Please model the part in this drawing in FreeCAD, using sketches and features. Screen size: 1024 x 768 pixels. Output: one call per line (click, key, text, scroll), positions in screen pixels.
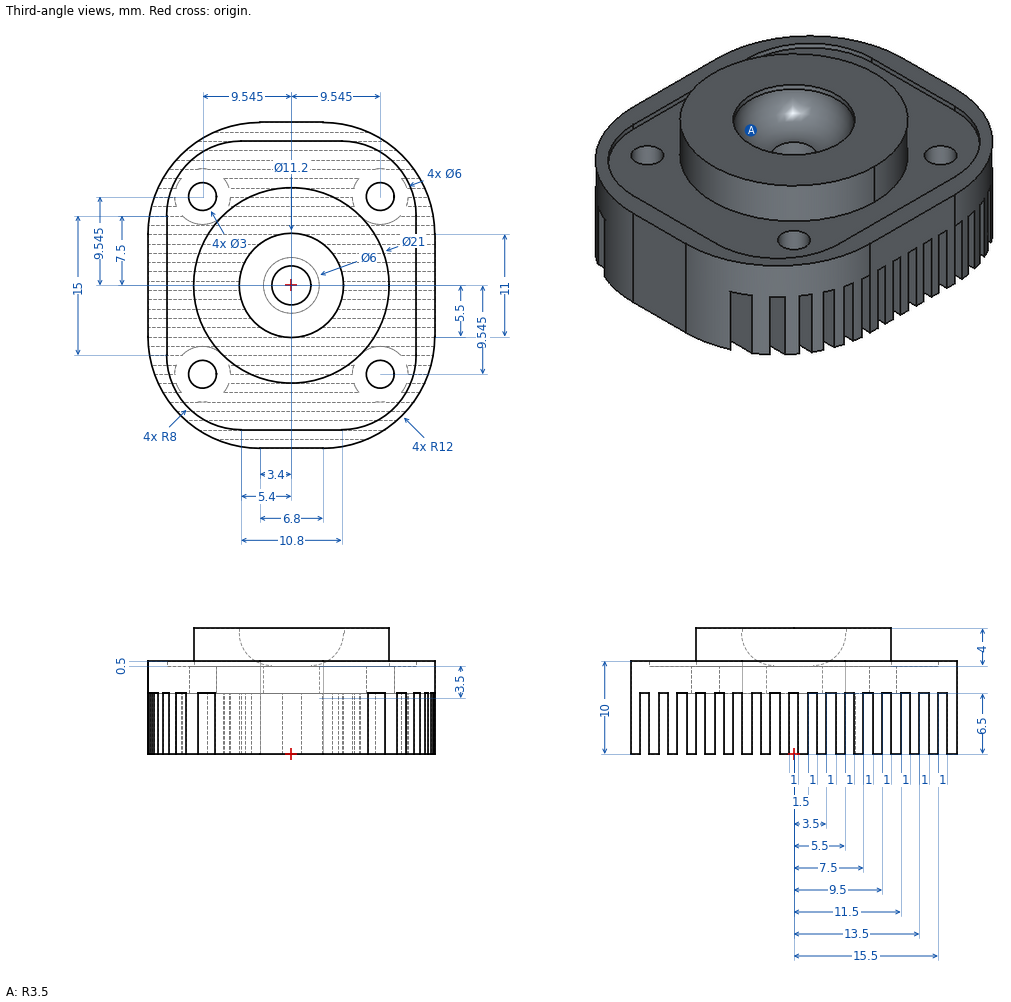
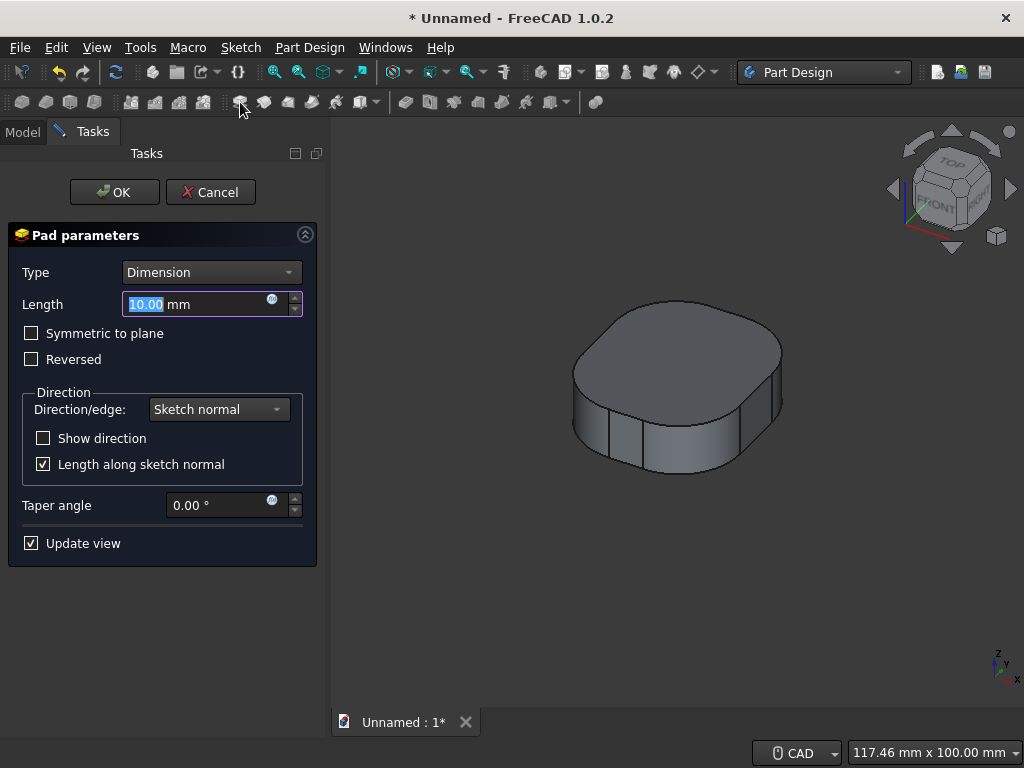
text(10)
key(Tab)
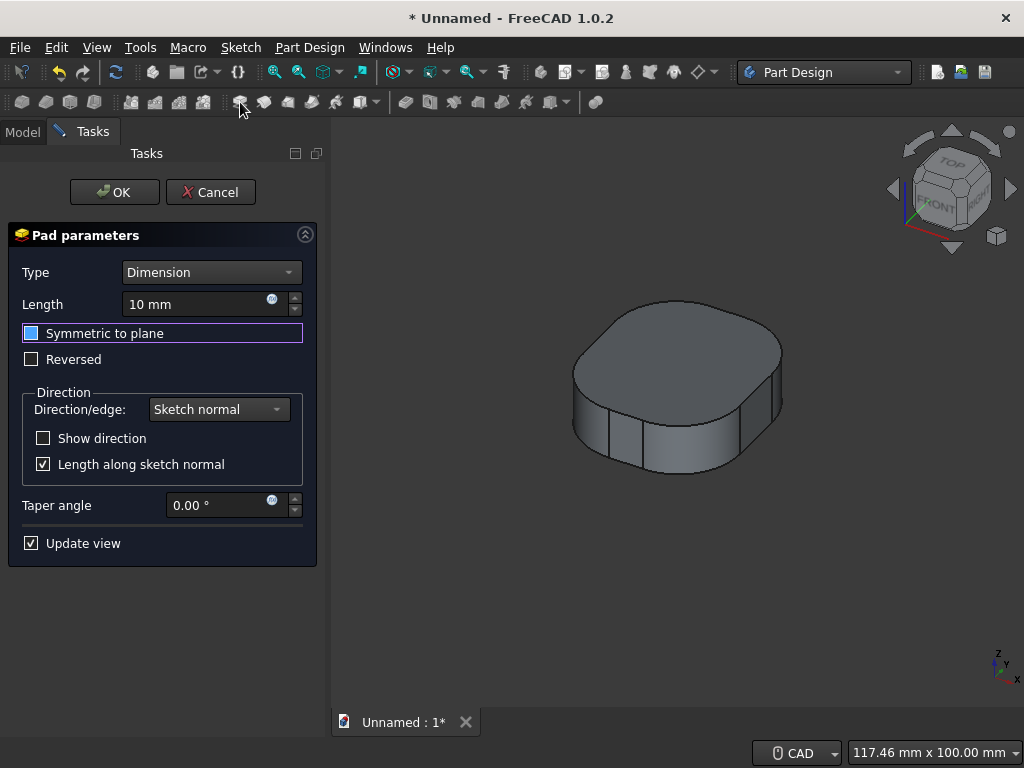
click(115, 192)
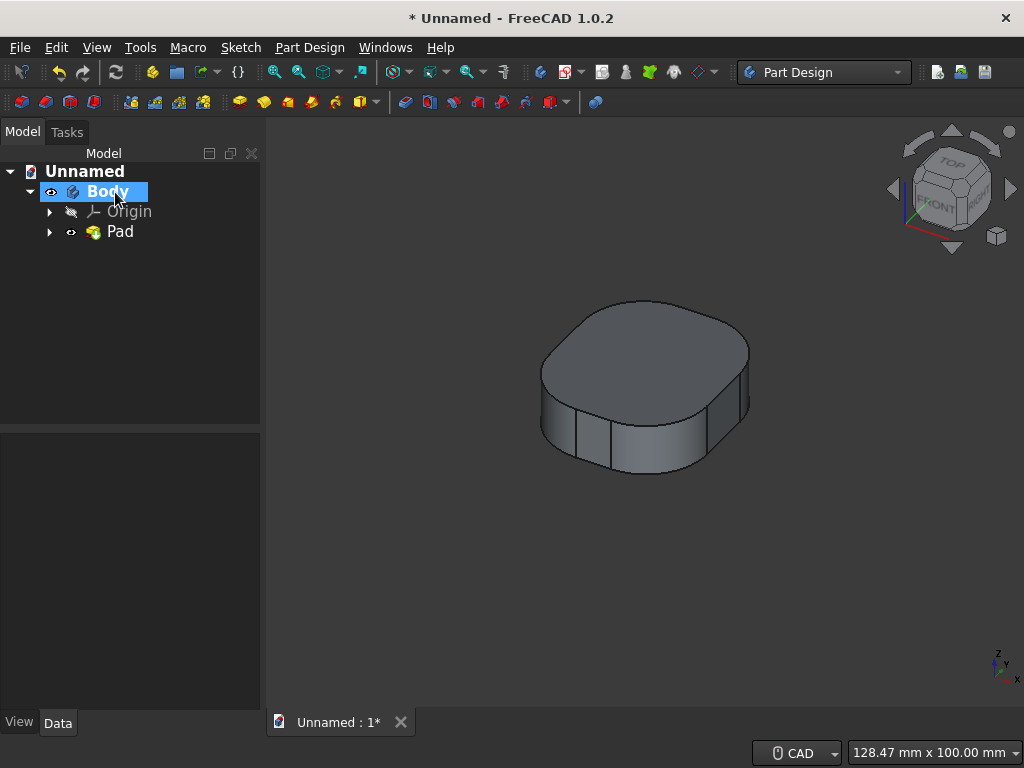
click(276, 72)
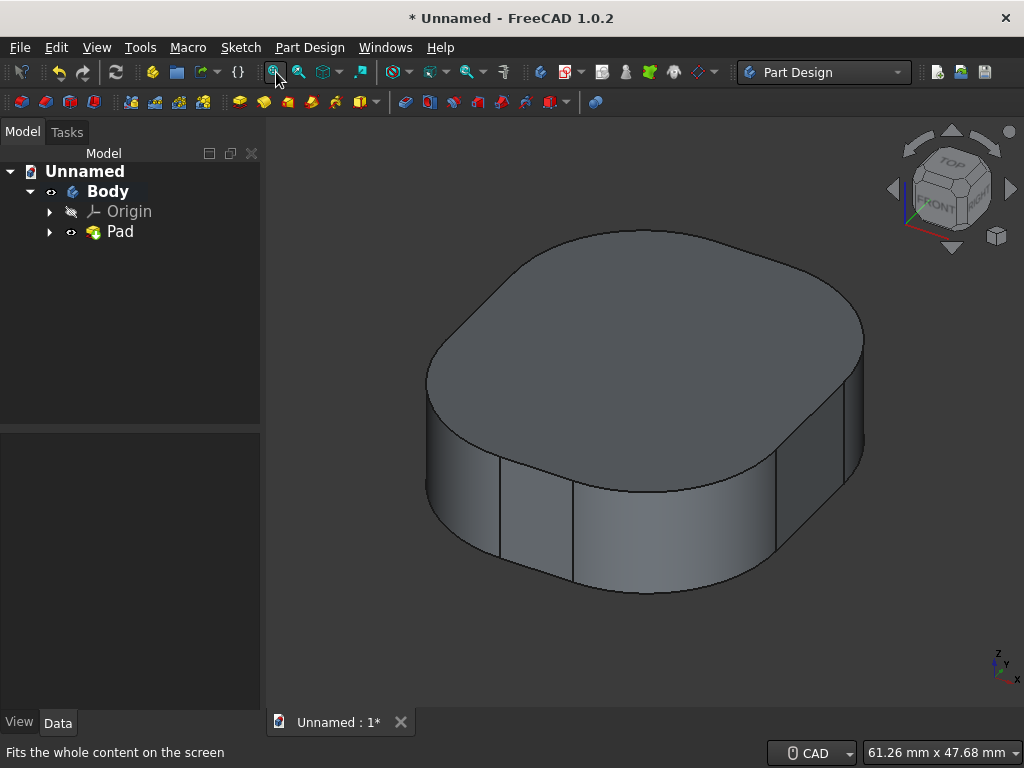
click(645, 360)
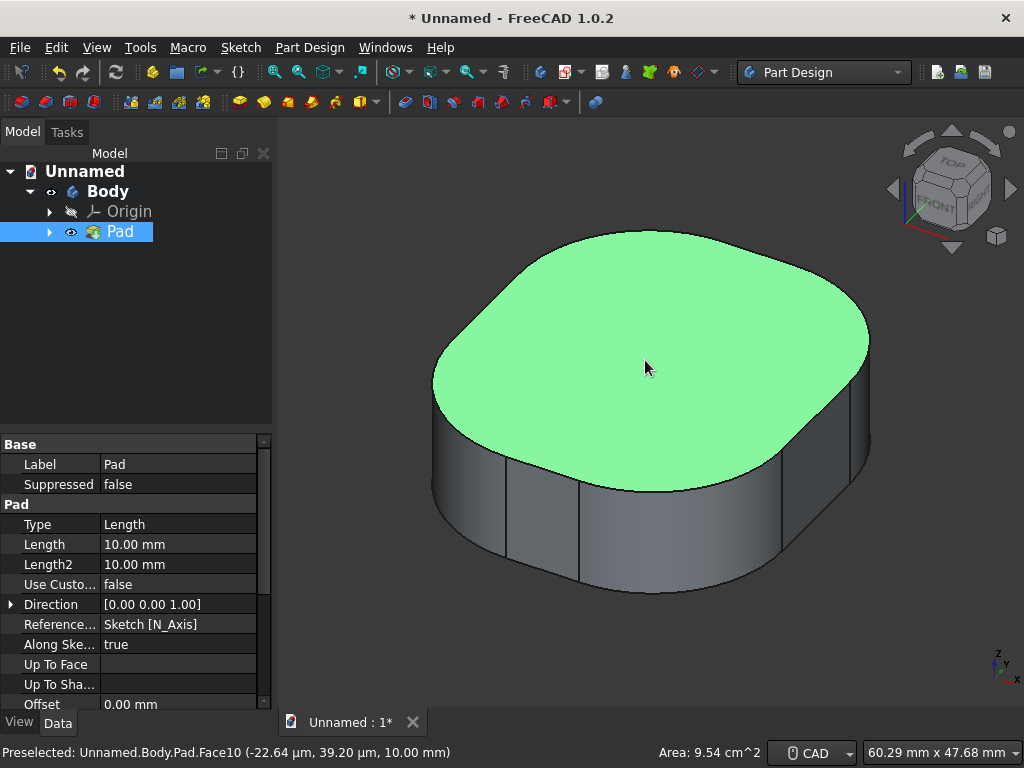
click(566, 72)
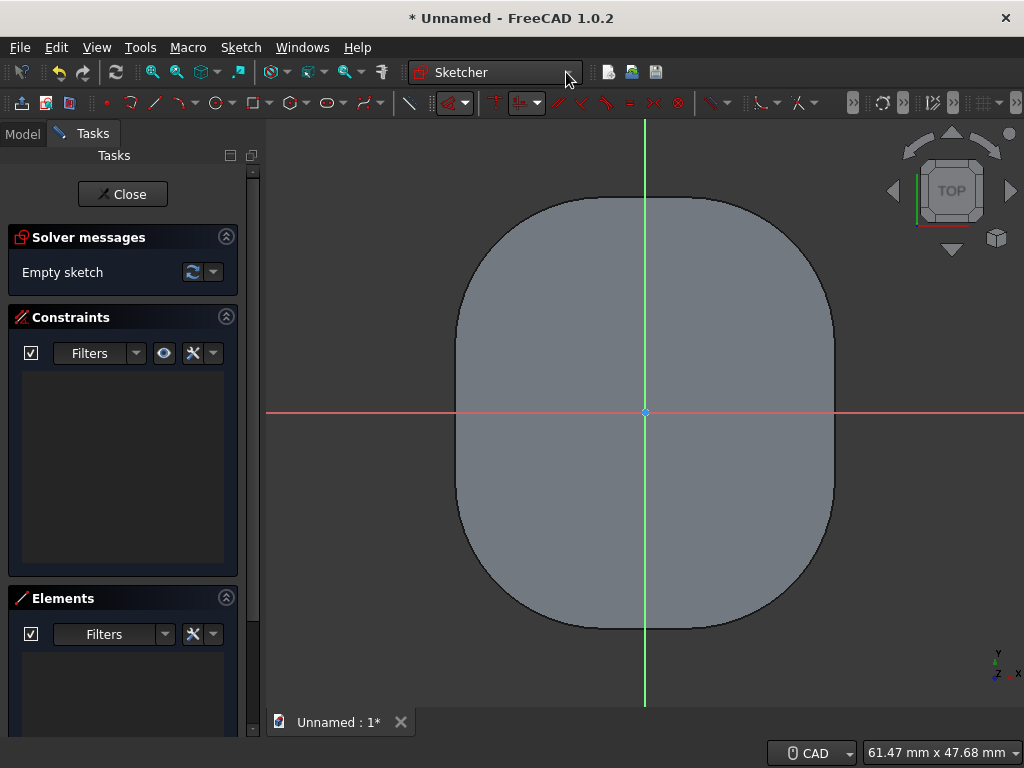
click(156, 104)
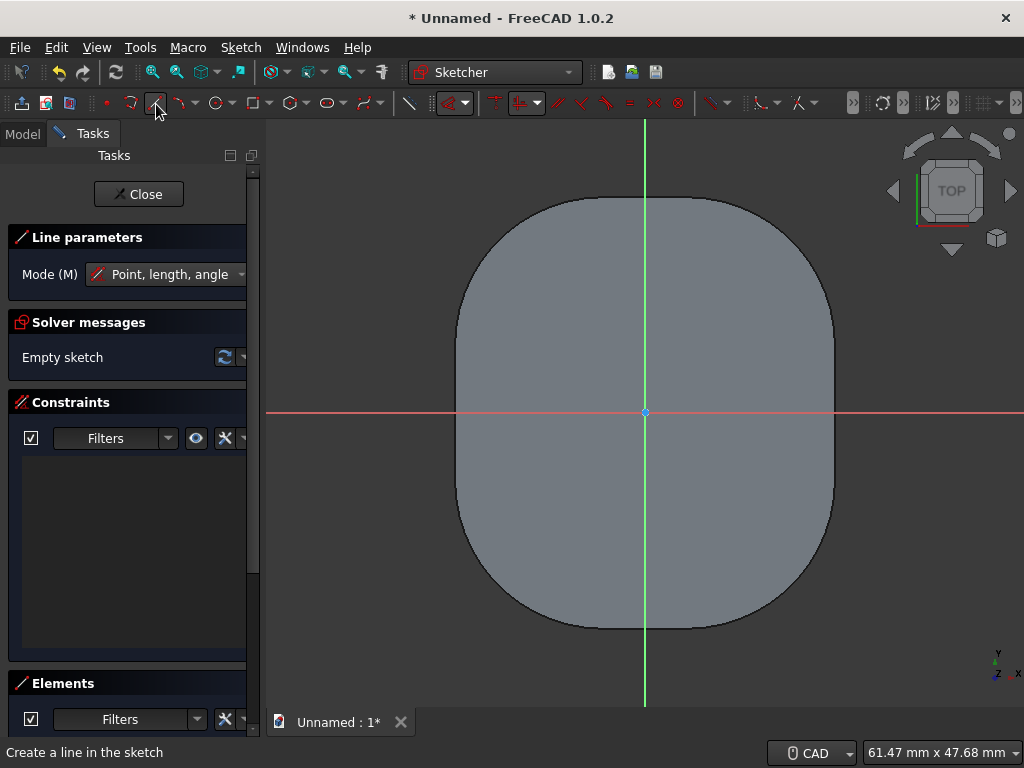
click(480, 321)
click(480, 505)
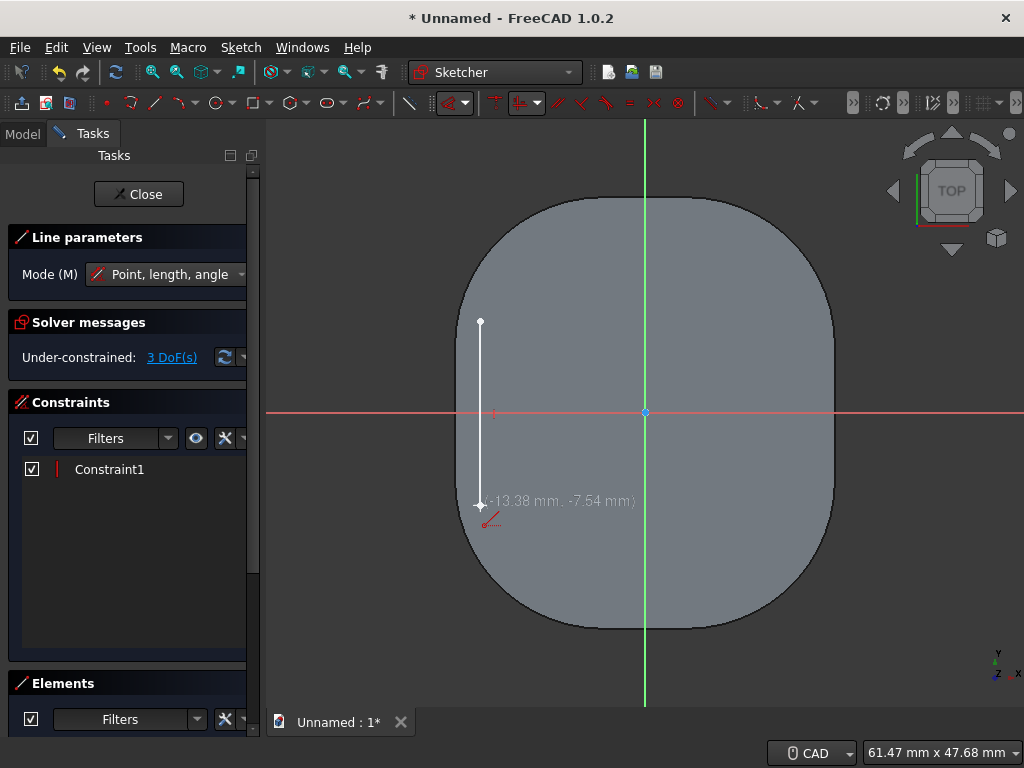
click(578, 604)
click(712, 604)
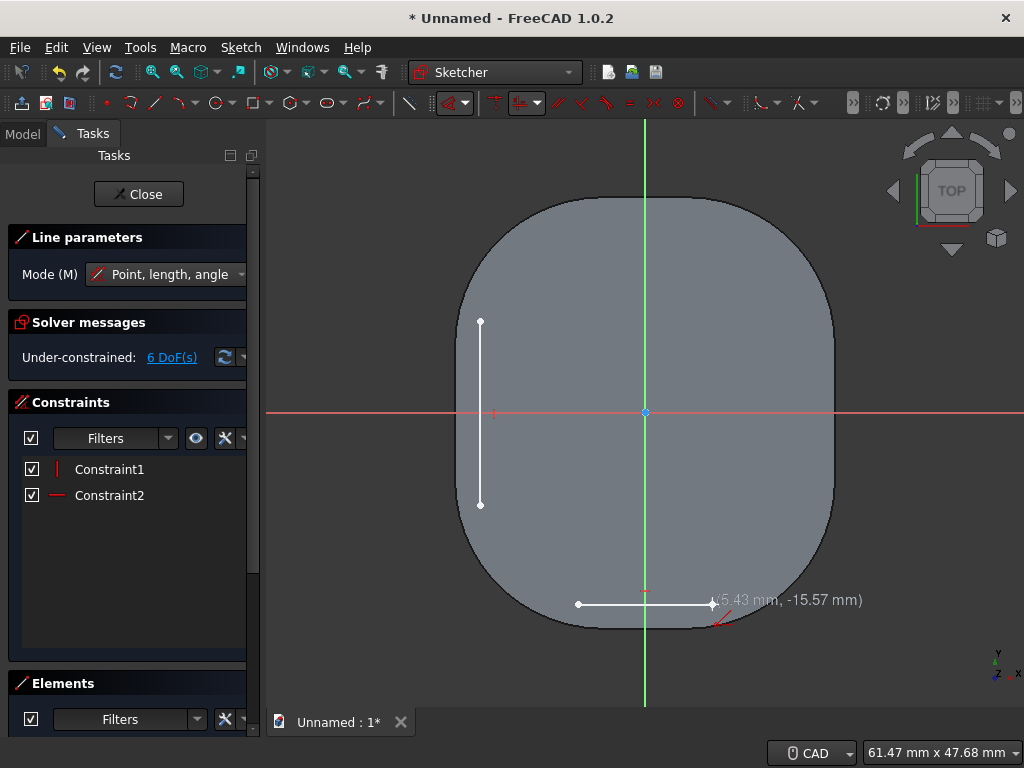
click(810, 505)
click(810, 321)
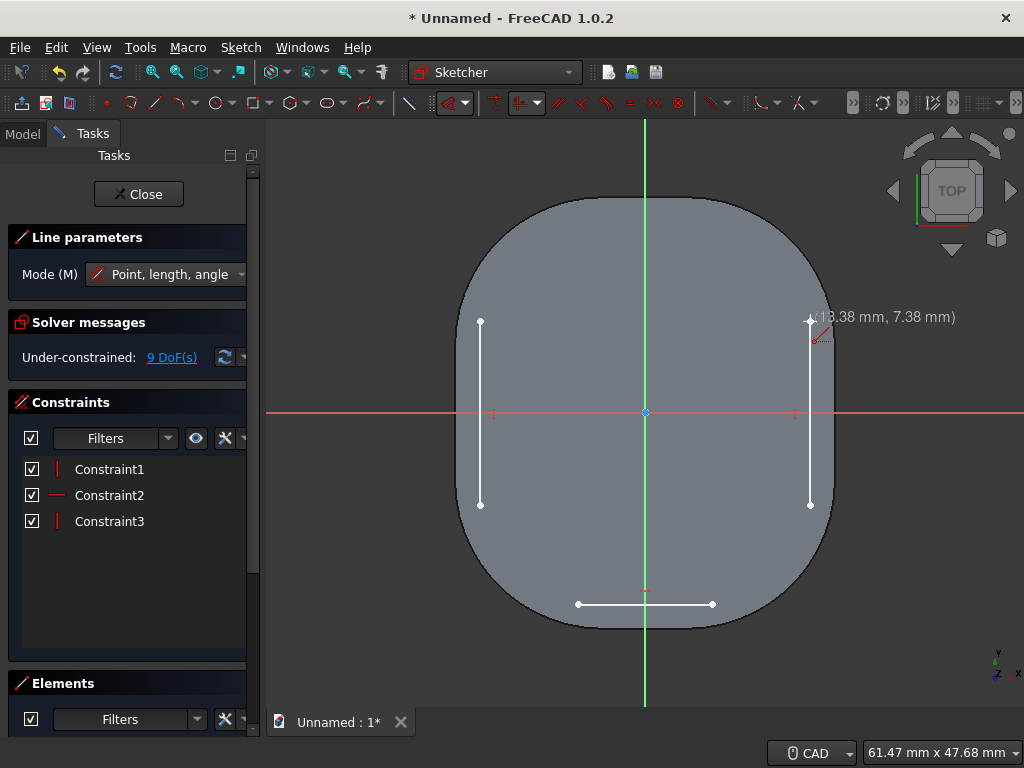
click(712, 222)
click(578, 222)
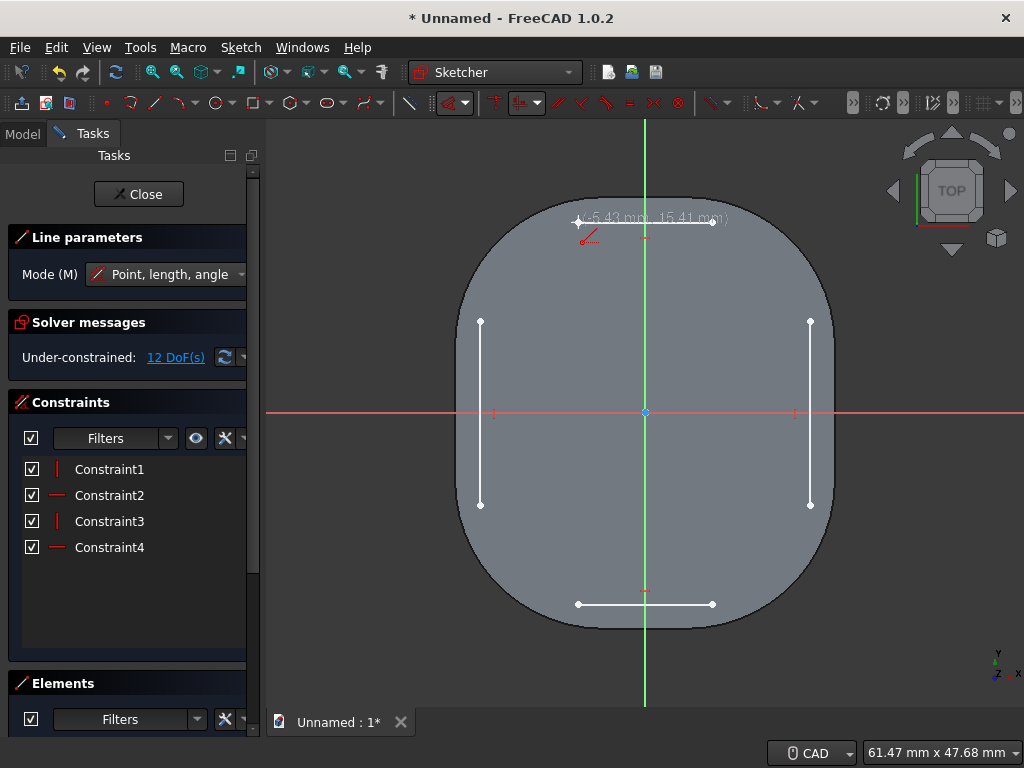
key(g)
key(3)
key(a)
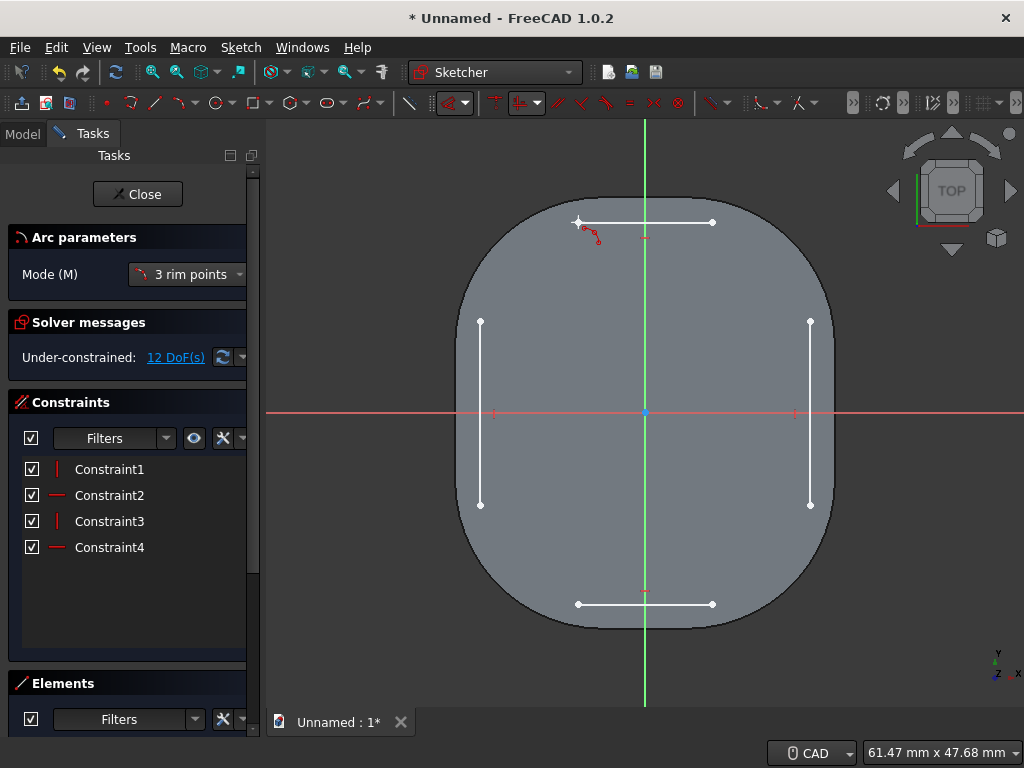
click(480, 506)
click(578, 605)
click(509, 575)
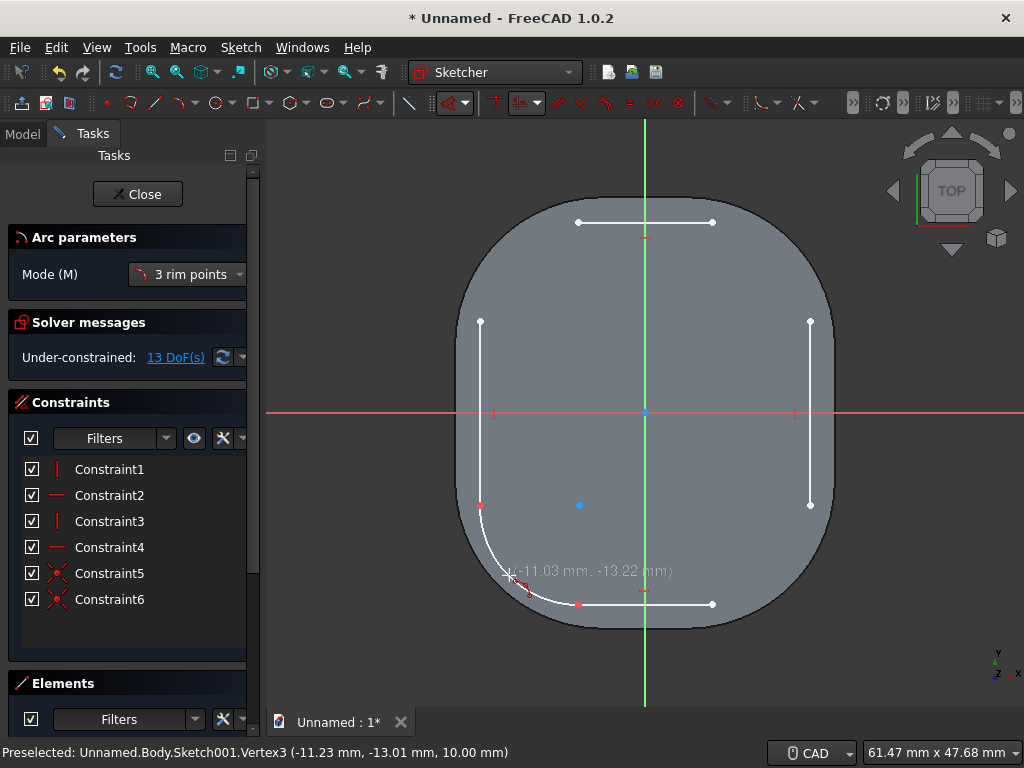
click(712, 605)
click(810, 506)
click(781, 575)